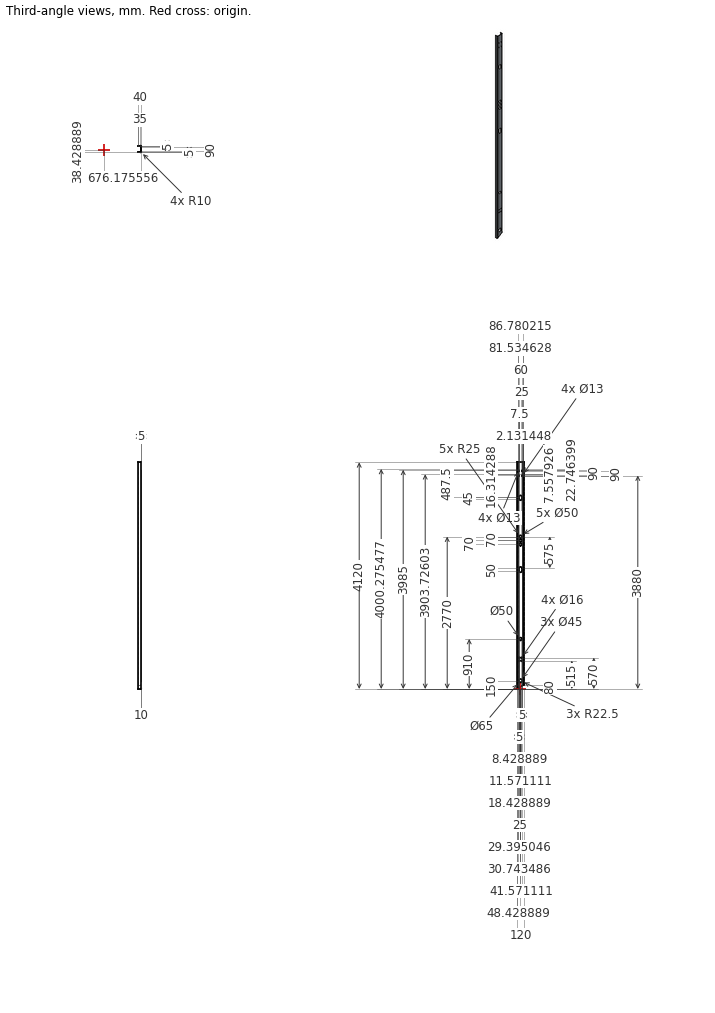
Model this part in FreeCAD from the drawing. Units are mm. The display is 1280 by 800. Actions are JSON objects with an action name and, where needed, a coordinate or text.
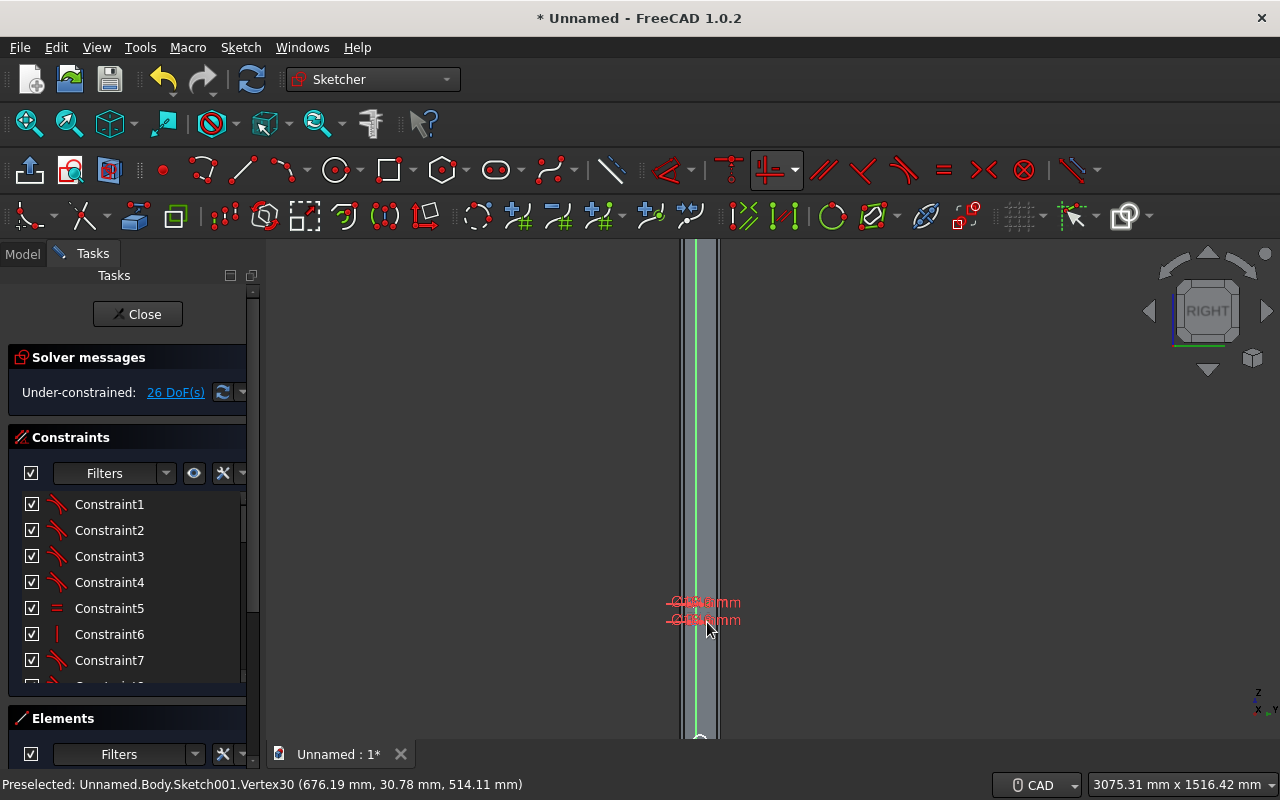
{"action": "key", "text": "v"}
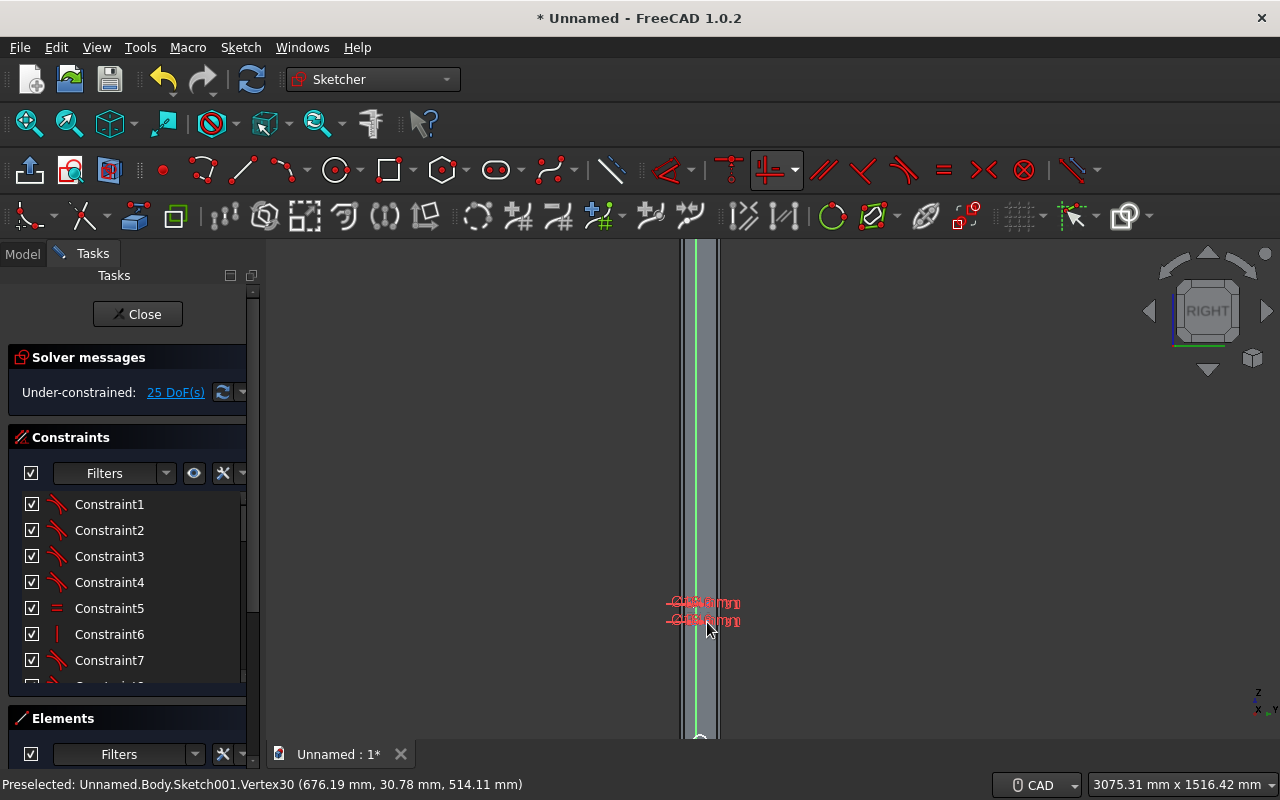
{"action": "left_click", "coordinate": [707, 605]}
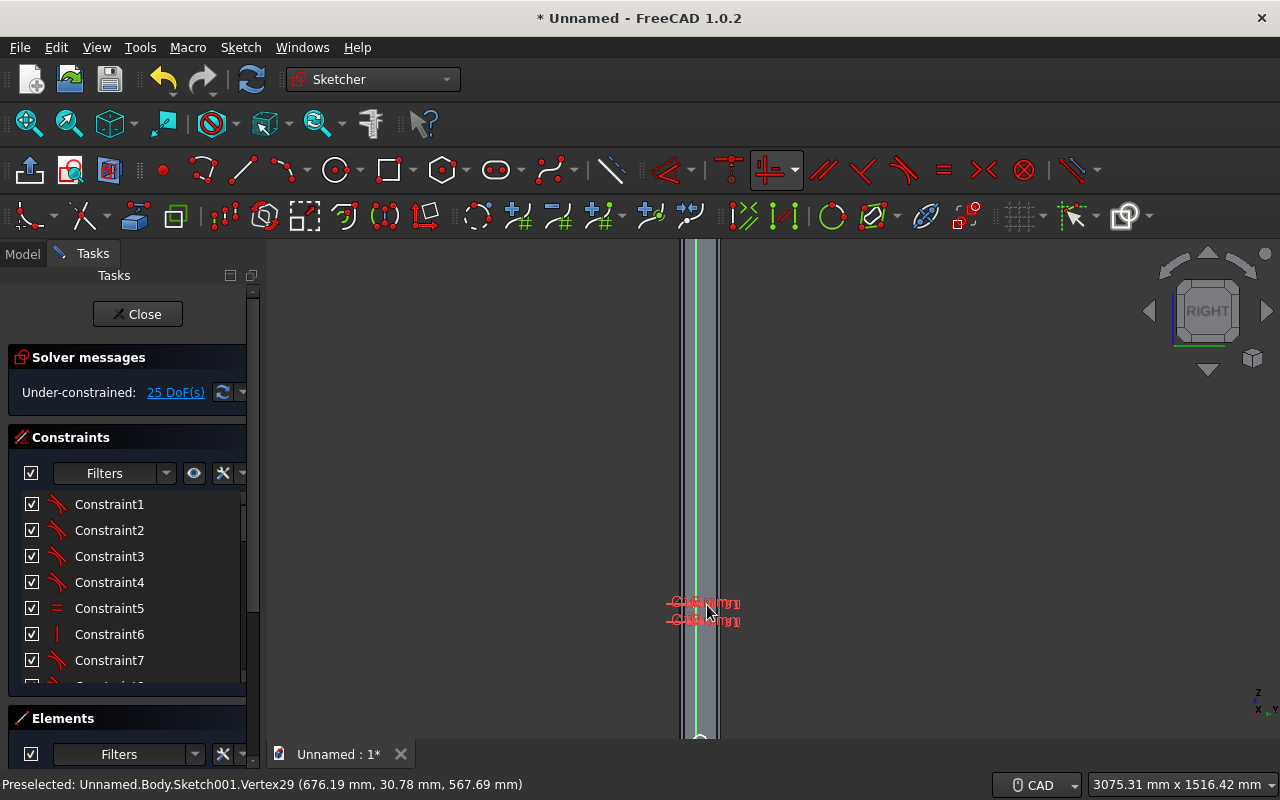
{"action": "left_click", "coordinate": [694, 604]}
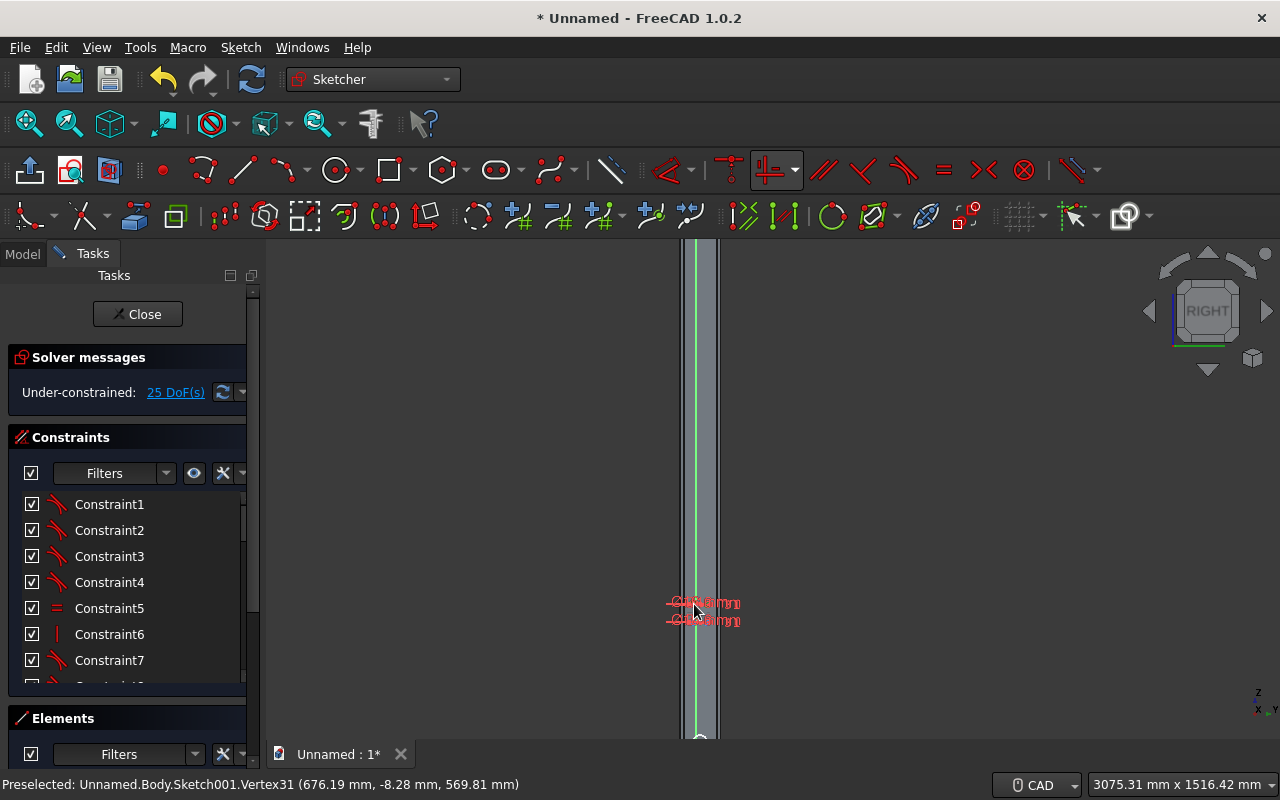
{"action": "key", "text": "h"}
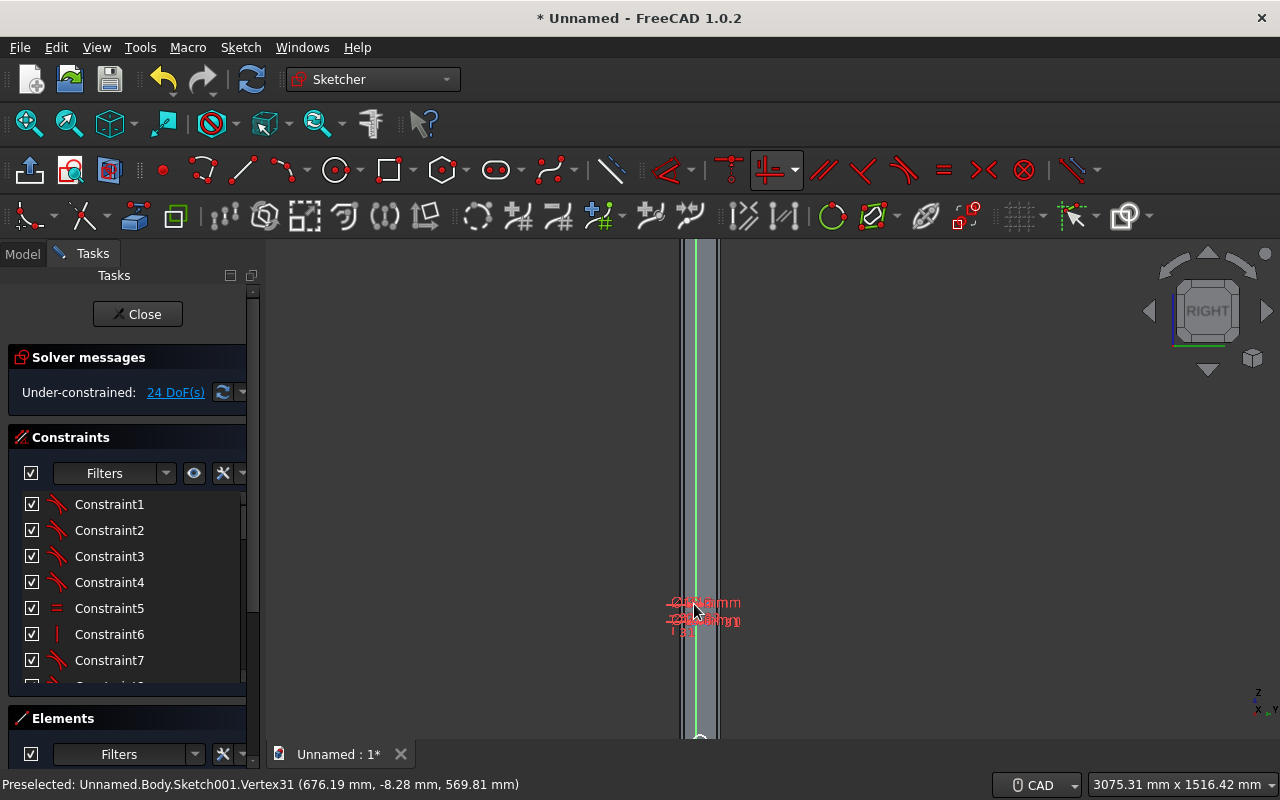
{"action": "left_click", "coordinate": [694, 605]}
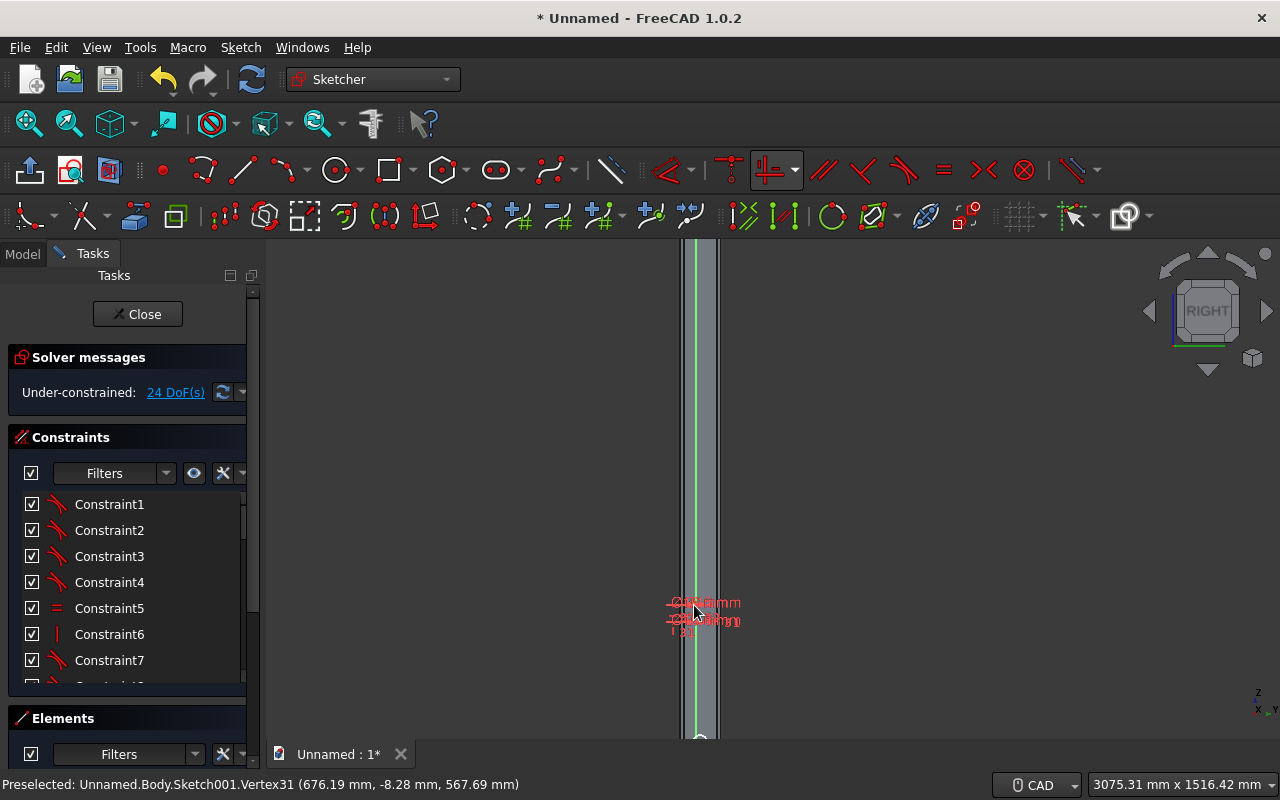
{"action": "scroll", "coordinate": [694, 622], "scroll_direction": "up", "scroll_amount": 4}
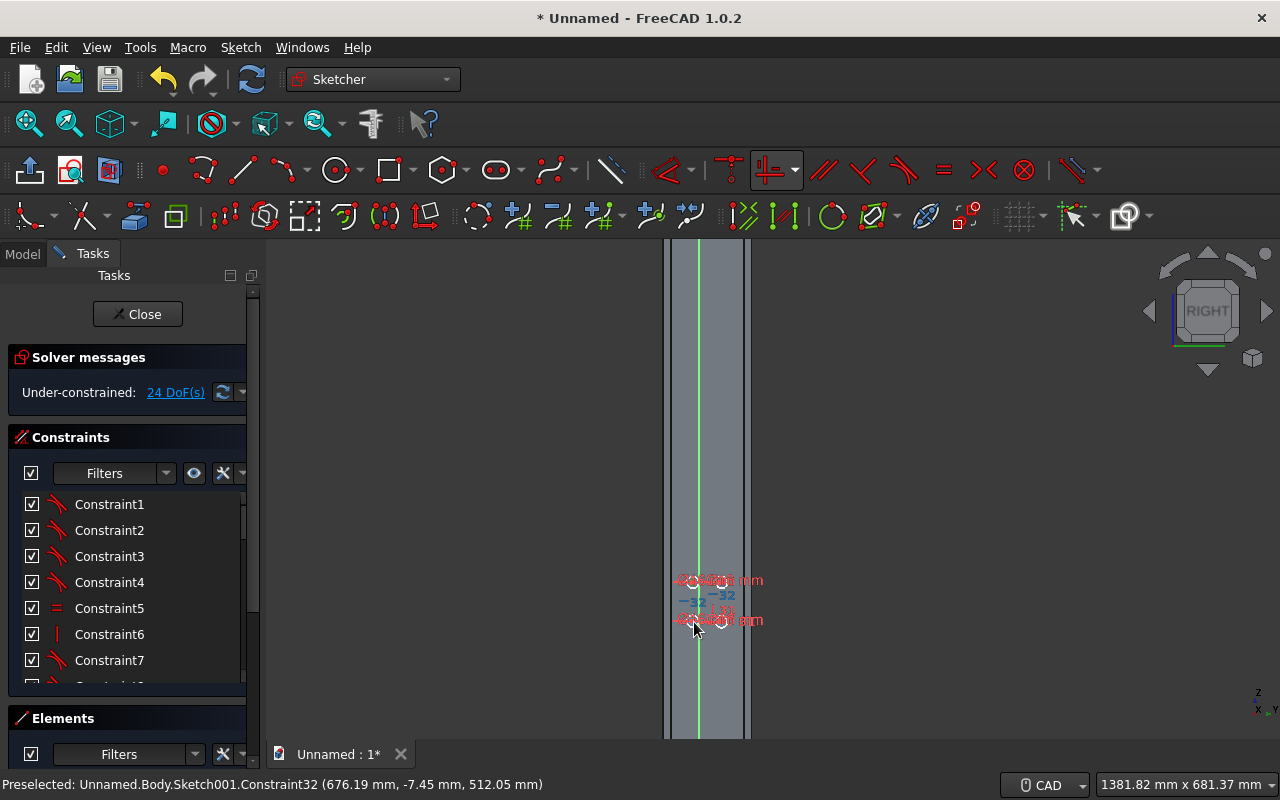
{"action": "left_click", "coordinate": [693, 621]}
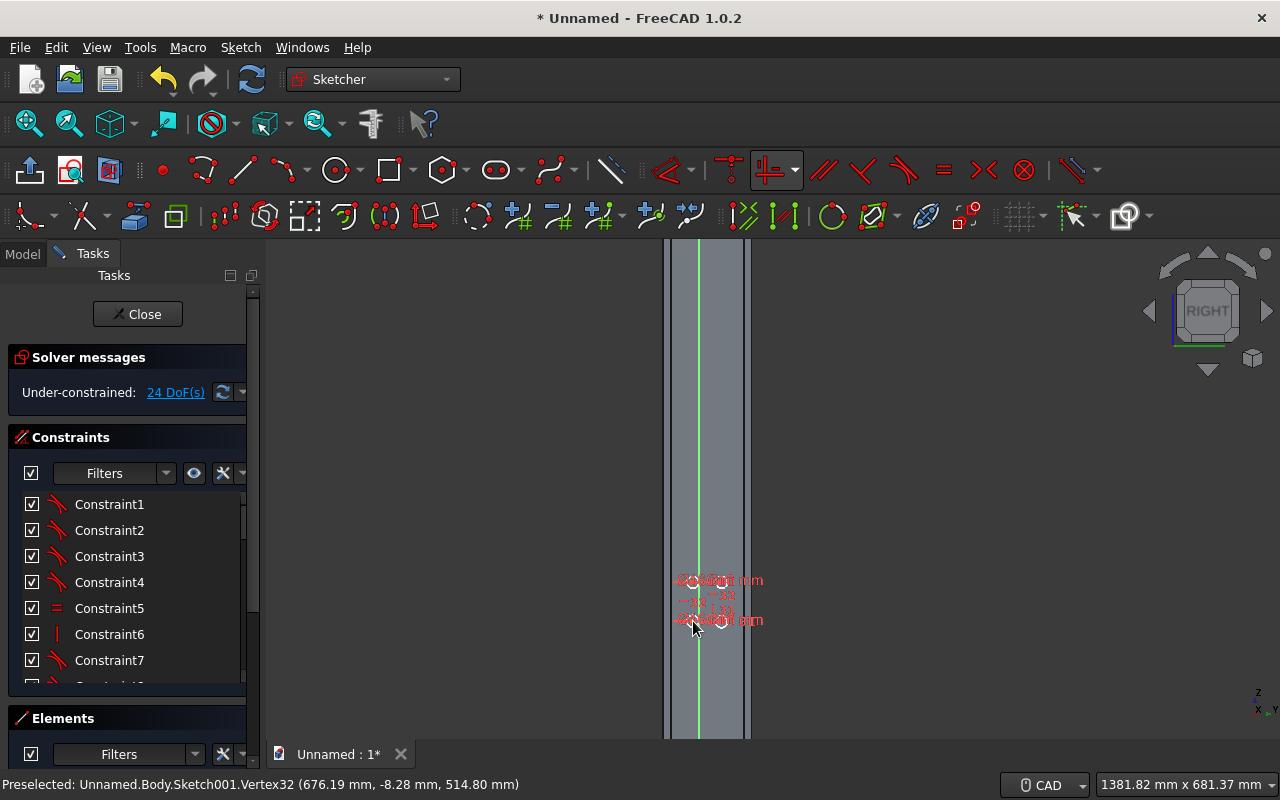
{"action": "key", "text": "v"}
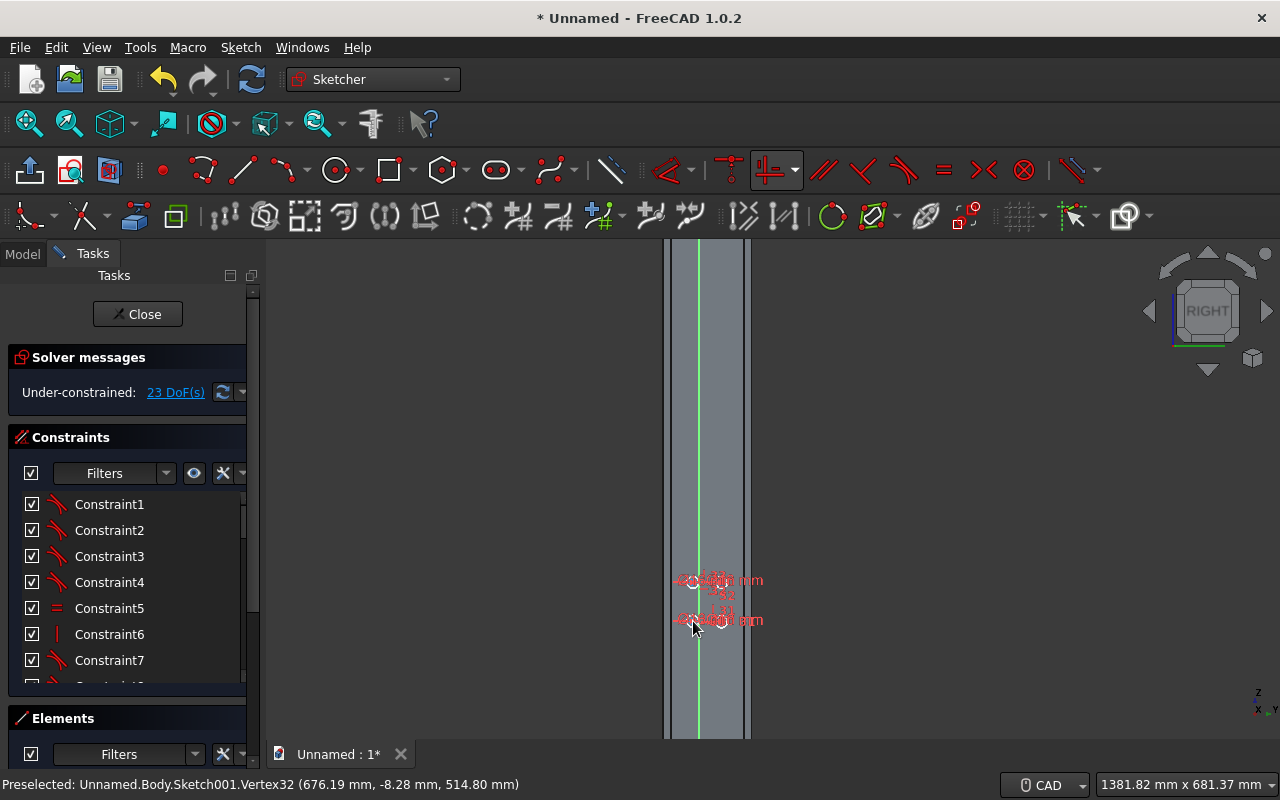
{"action": "scroll", "coordinate": [722, 622], "scroll_direction": "up", "scroll_amount": 4}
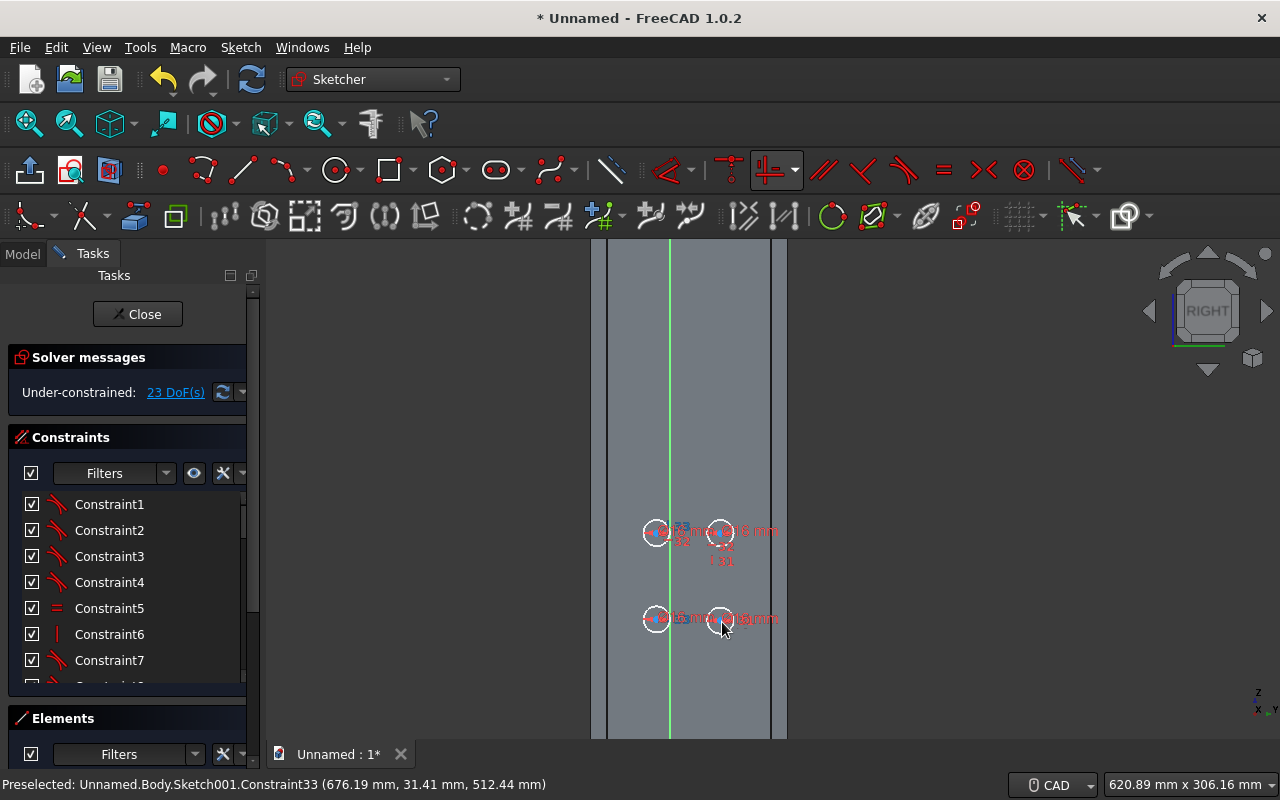
{"action": "left_click", "coordinate": [720, 621]}